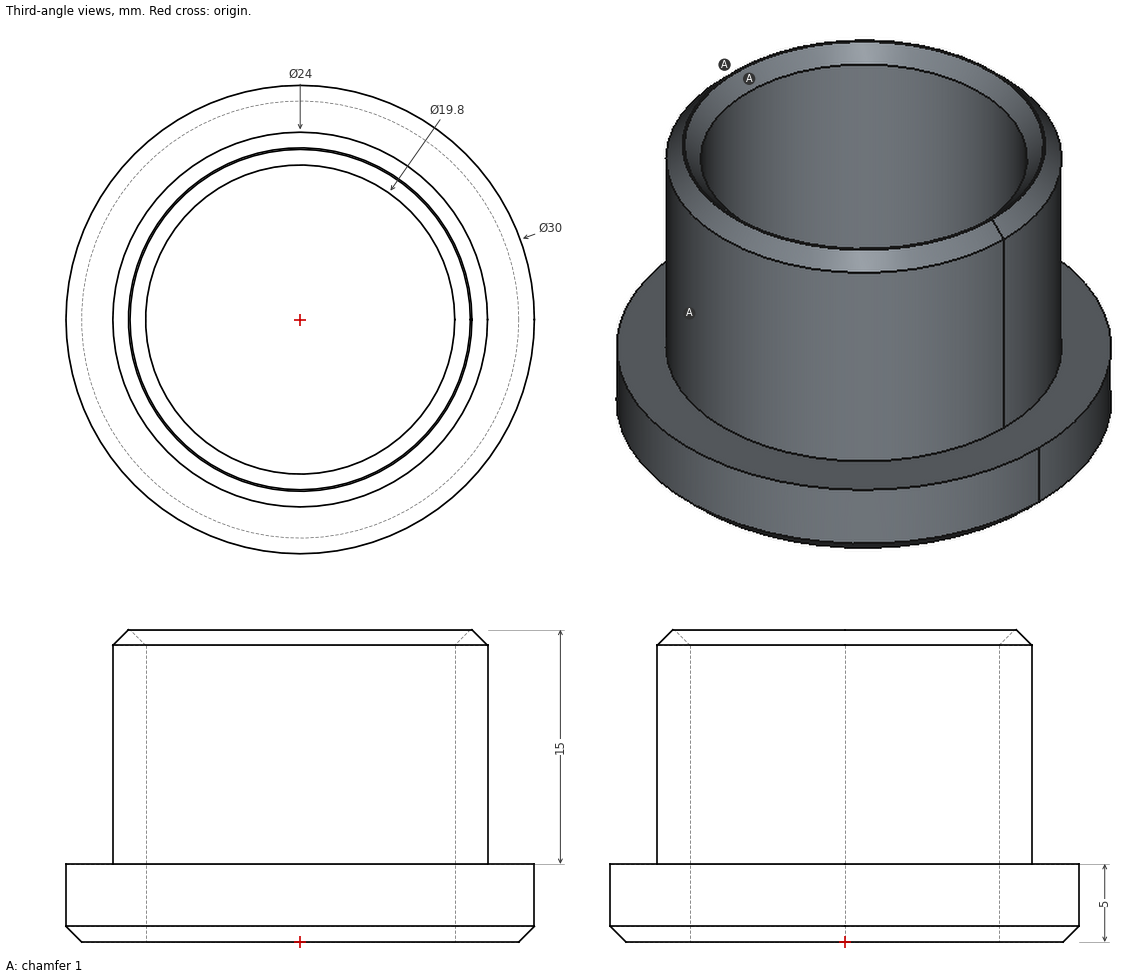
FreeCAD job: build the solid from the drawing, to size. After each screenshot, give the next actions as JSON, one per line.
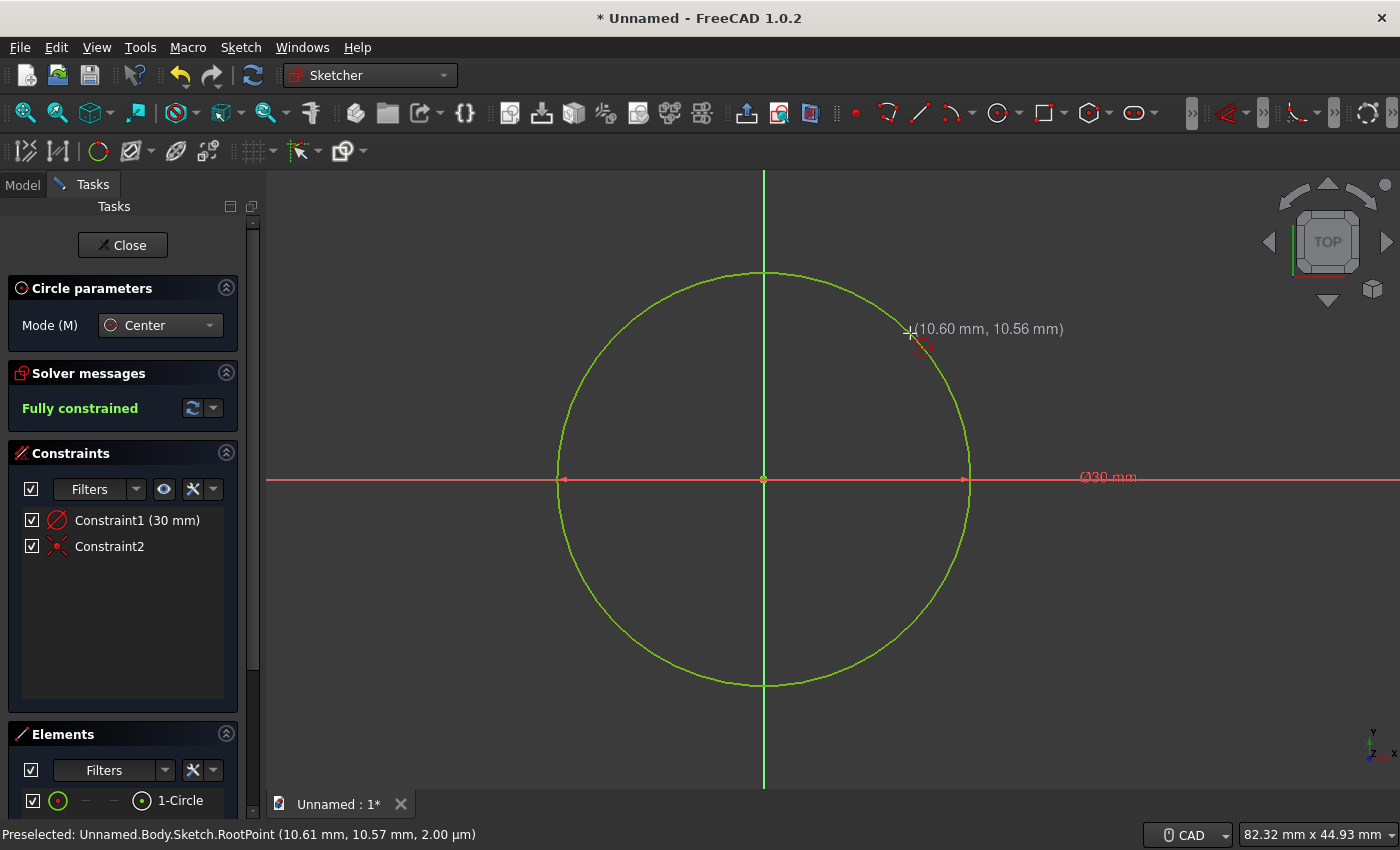
{"action": "left_click", "coordinate": [764, 480]}
{"action": "mouse_move", "coordinate": [860, 383]}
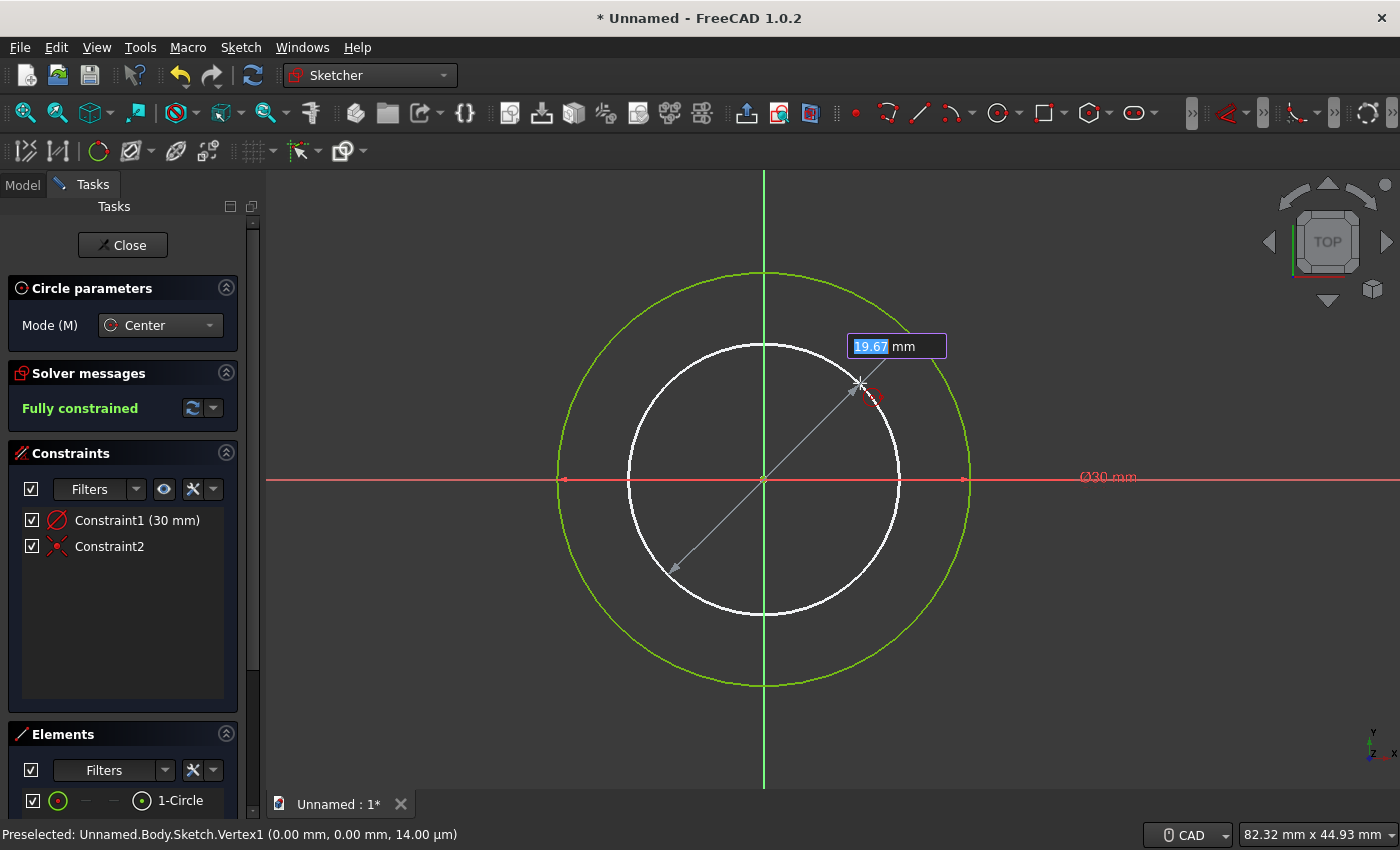
{"action": "type", "text": "19.8"}
{"action": "key", "text": "Return"}
{"action": "key", "text": "Escape"}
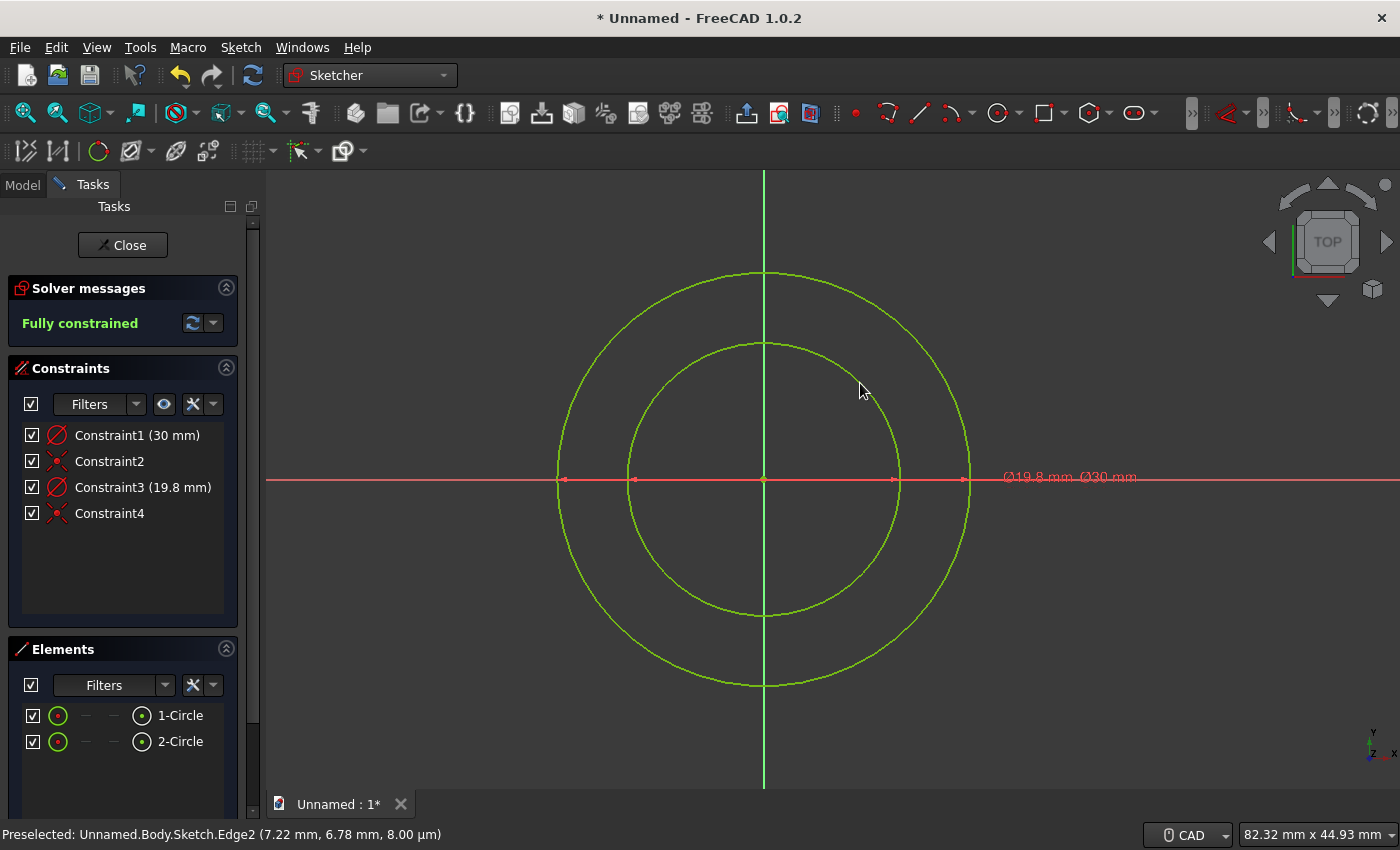
{"action": "left_click", "coordinate": [123, 245]}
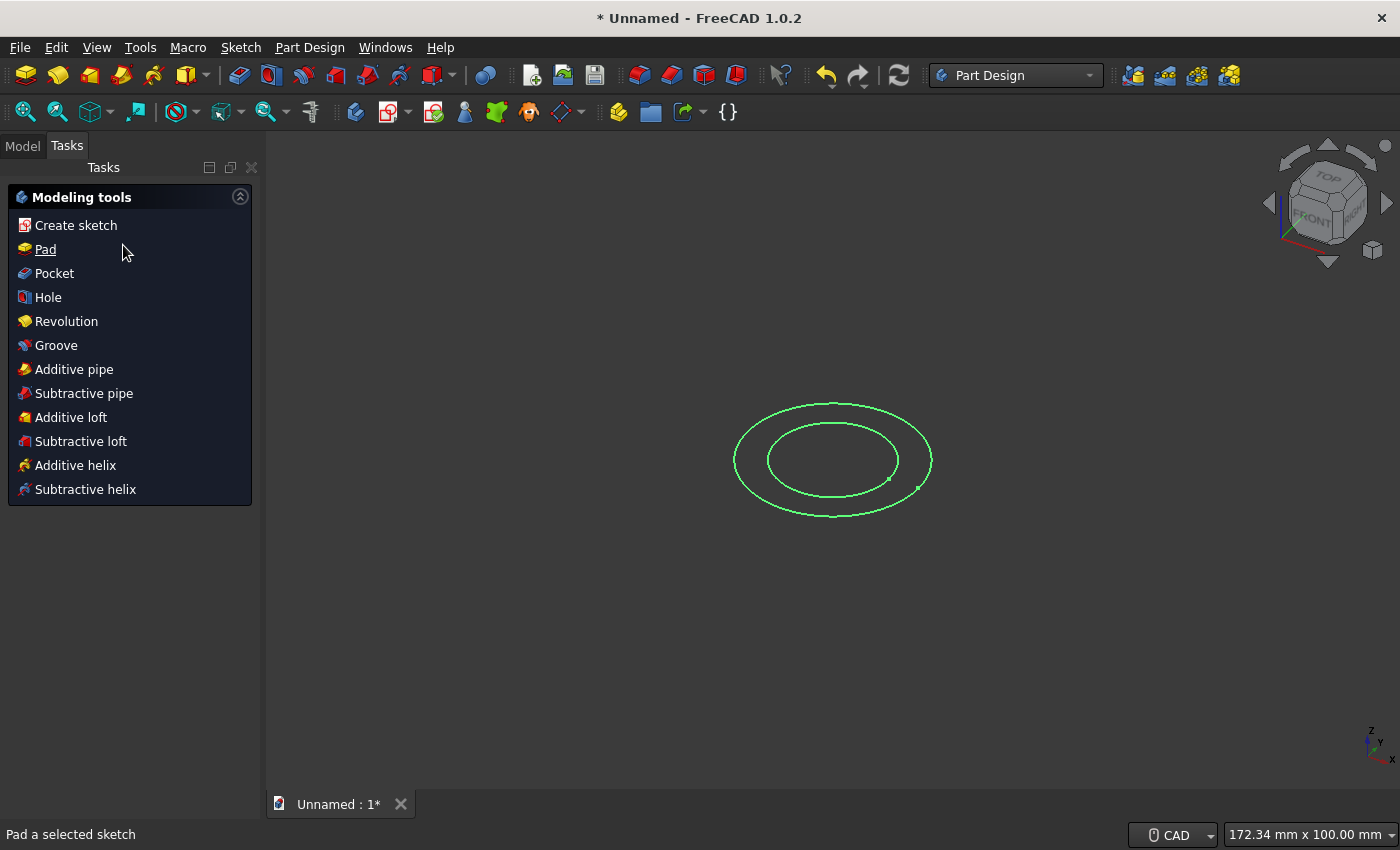
{"action": "left_click", "coordinate": [26, 76]}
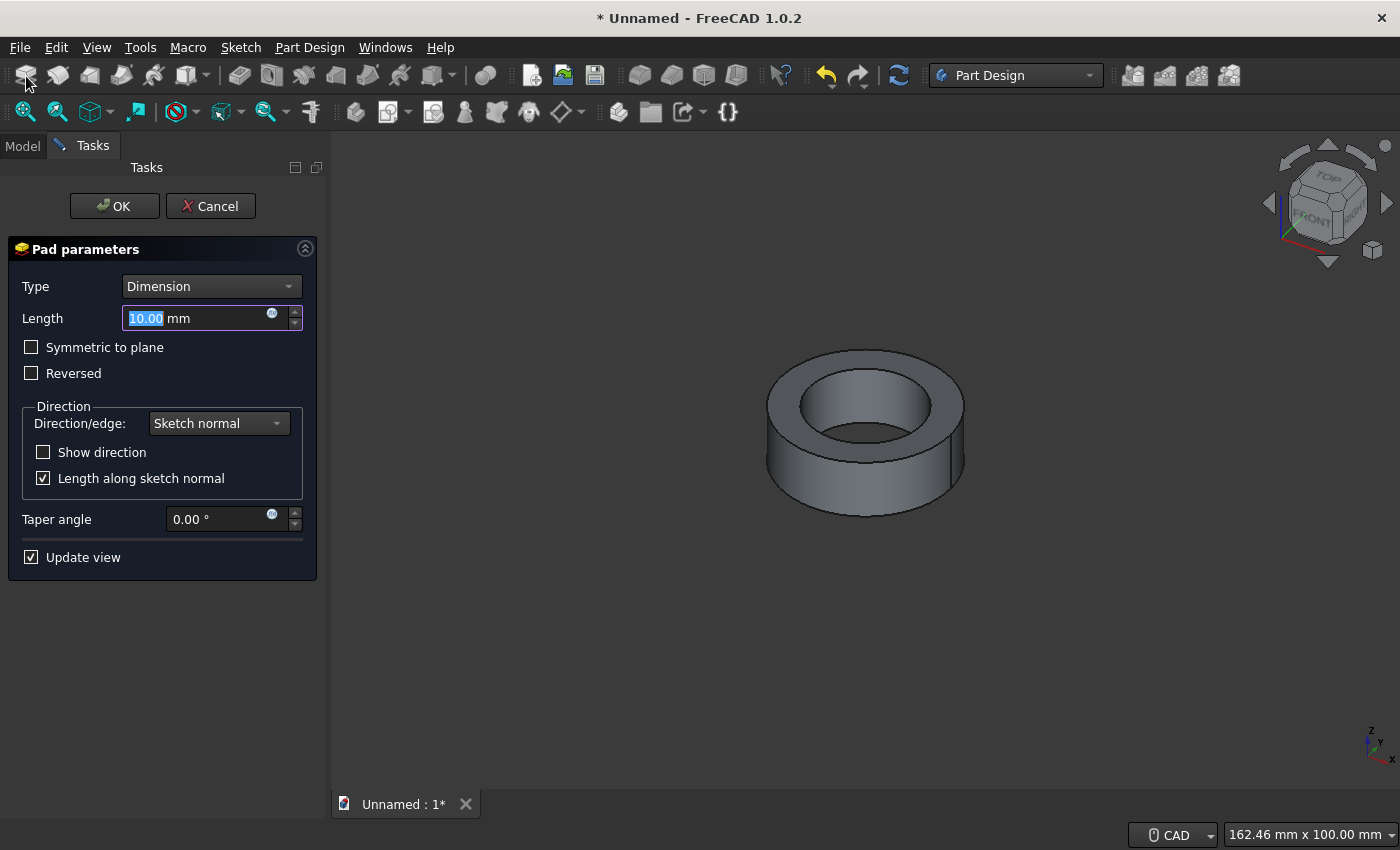
{"action": "type", "text": "5"}
{"action": "key", "text": "Tab"}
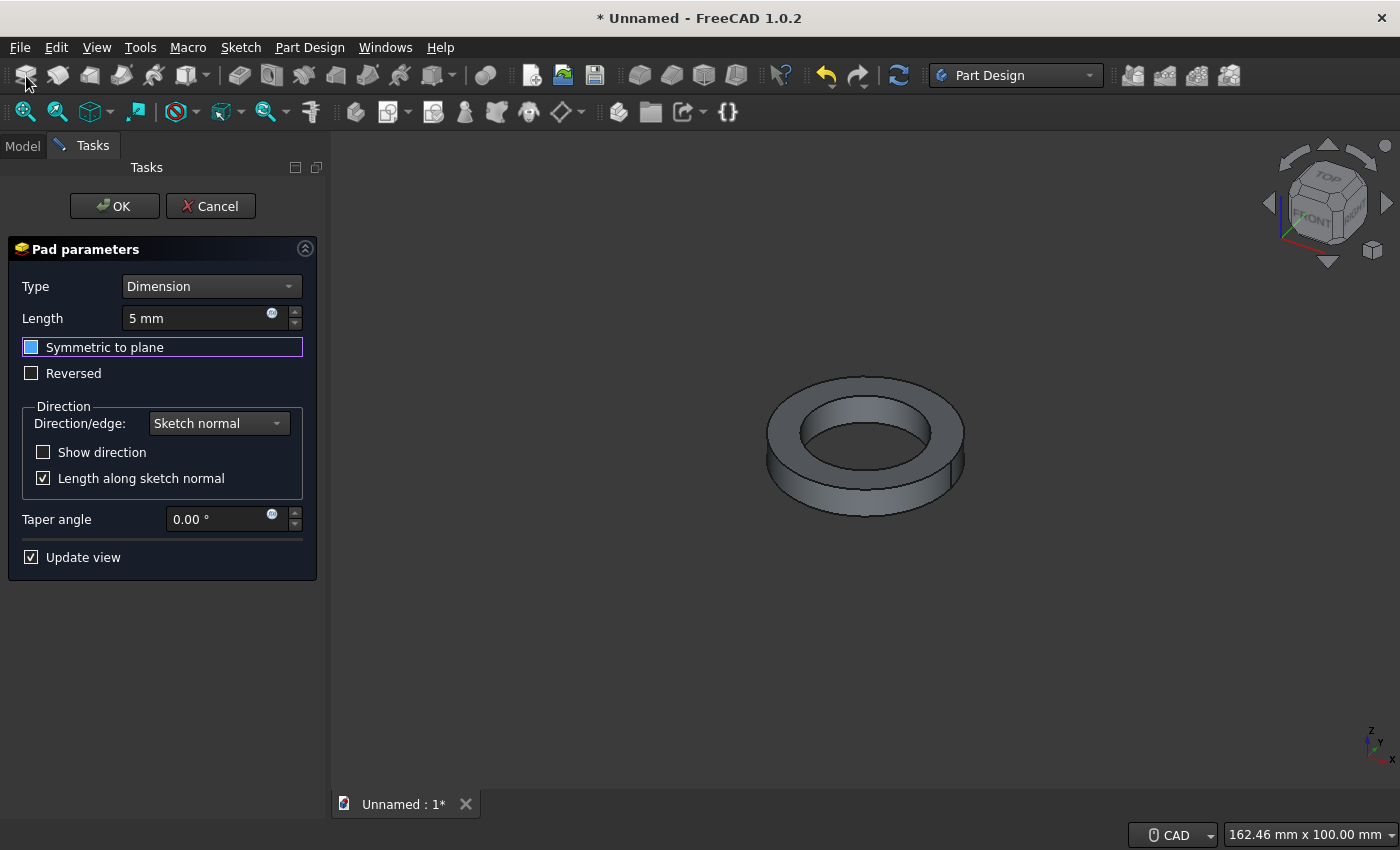
{"action": "left_click", "coordinate": [115, 206]}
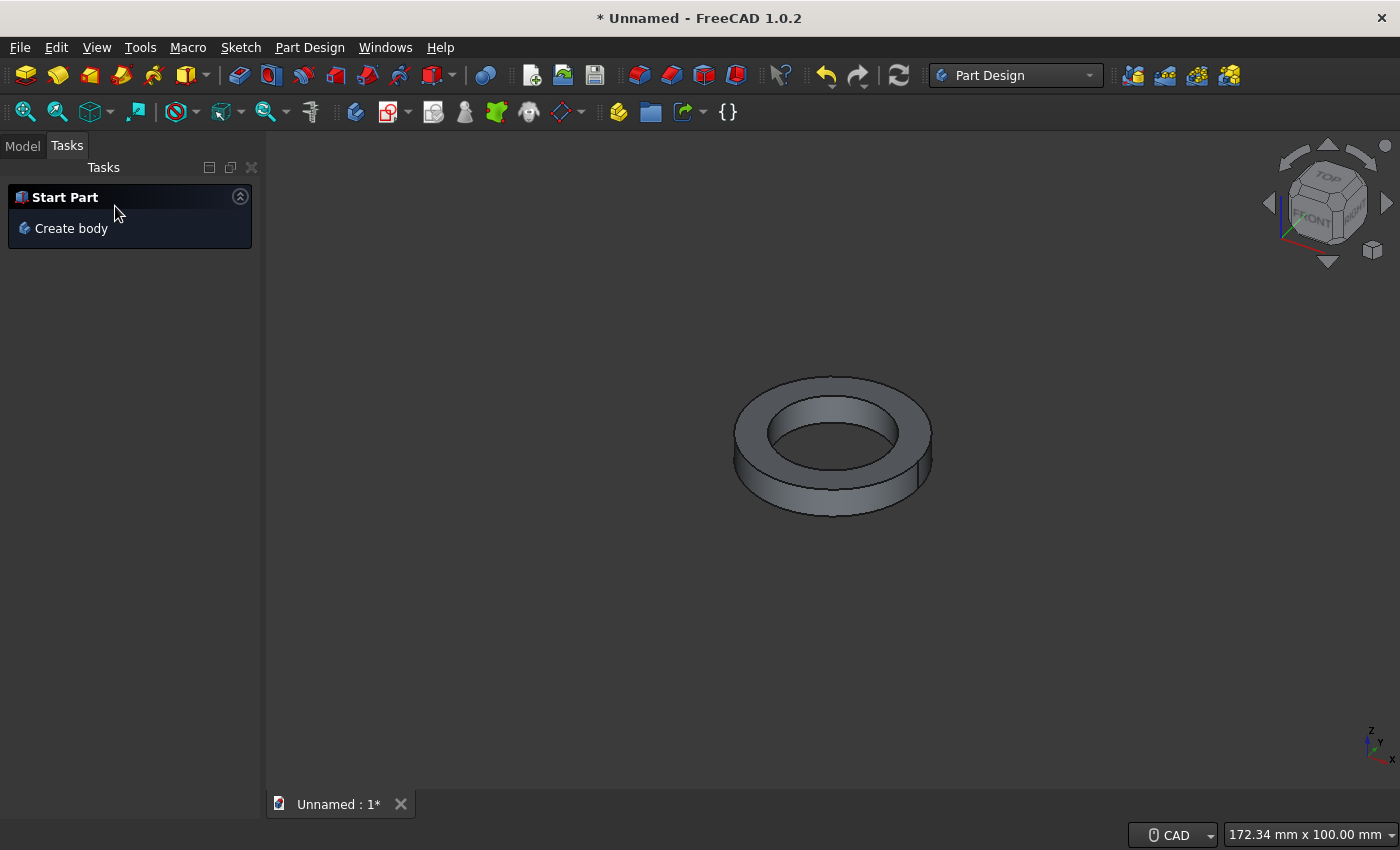
{"action": "key", "text": "v f"}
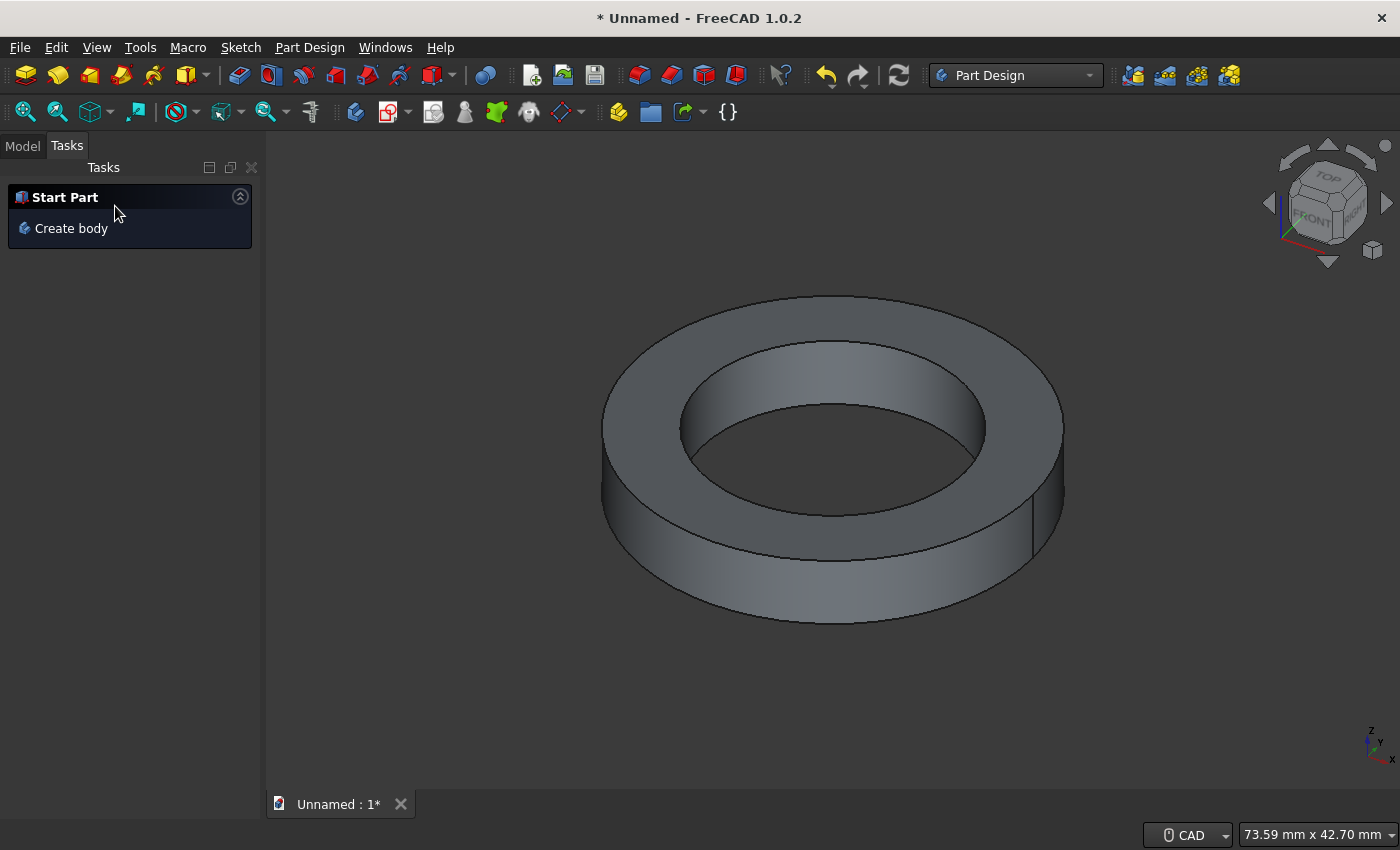
{"action": "left_click", "coordinate": [1013, 400]}